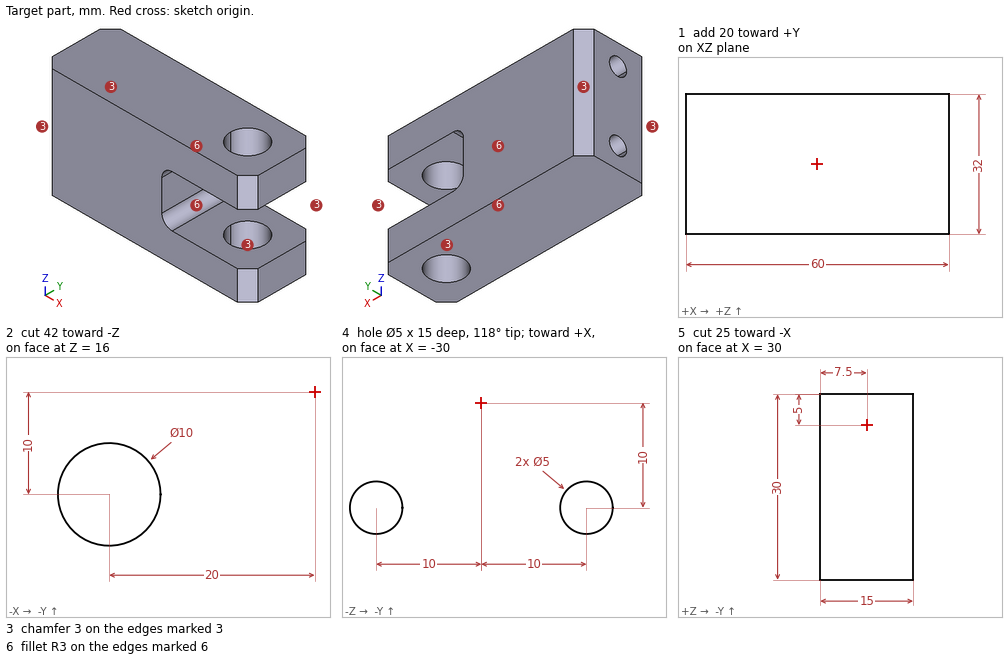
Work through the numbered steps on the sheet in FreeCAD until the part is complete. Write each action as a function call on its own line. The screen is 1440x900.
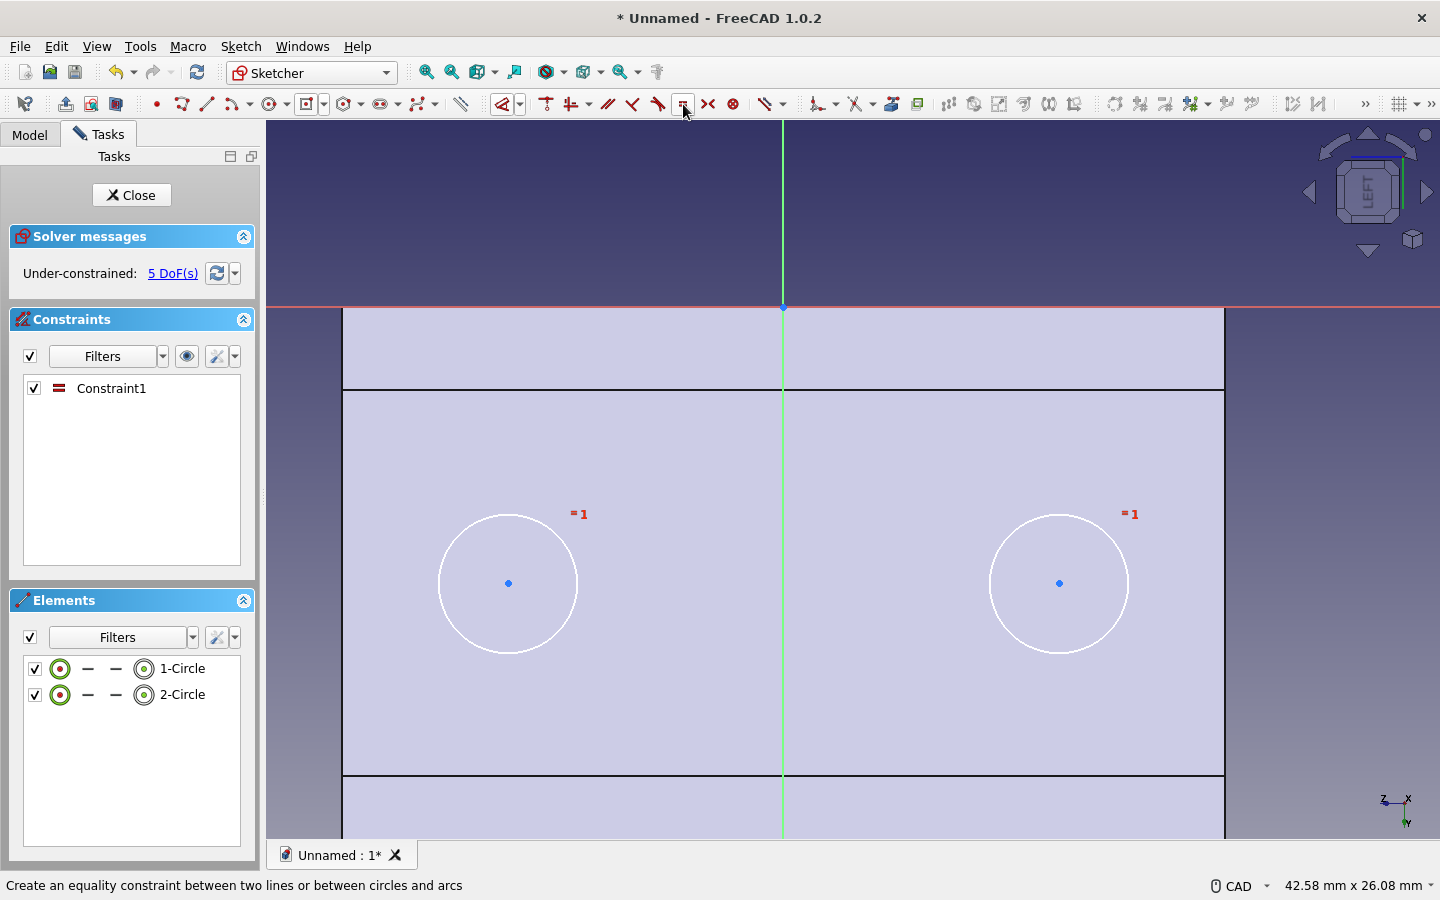
click(1059, 584)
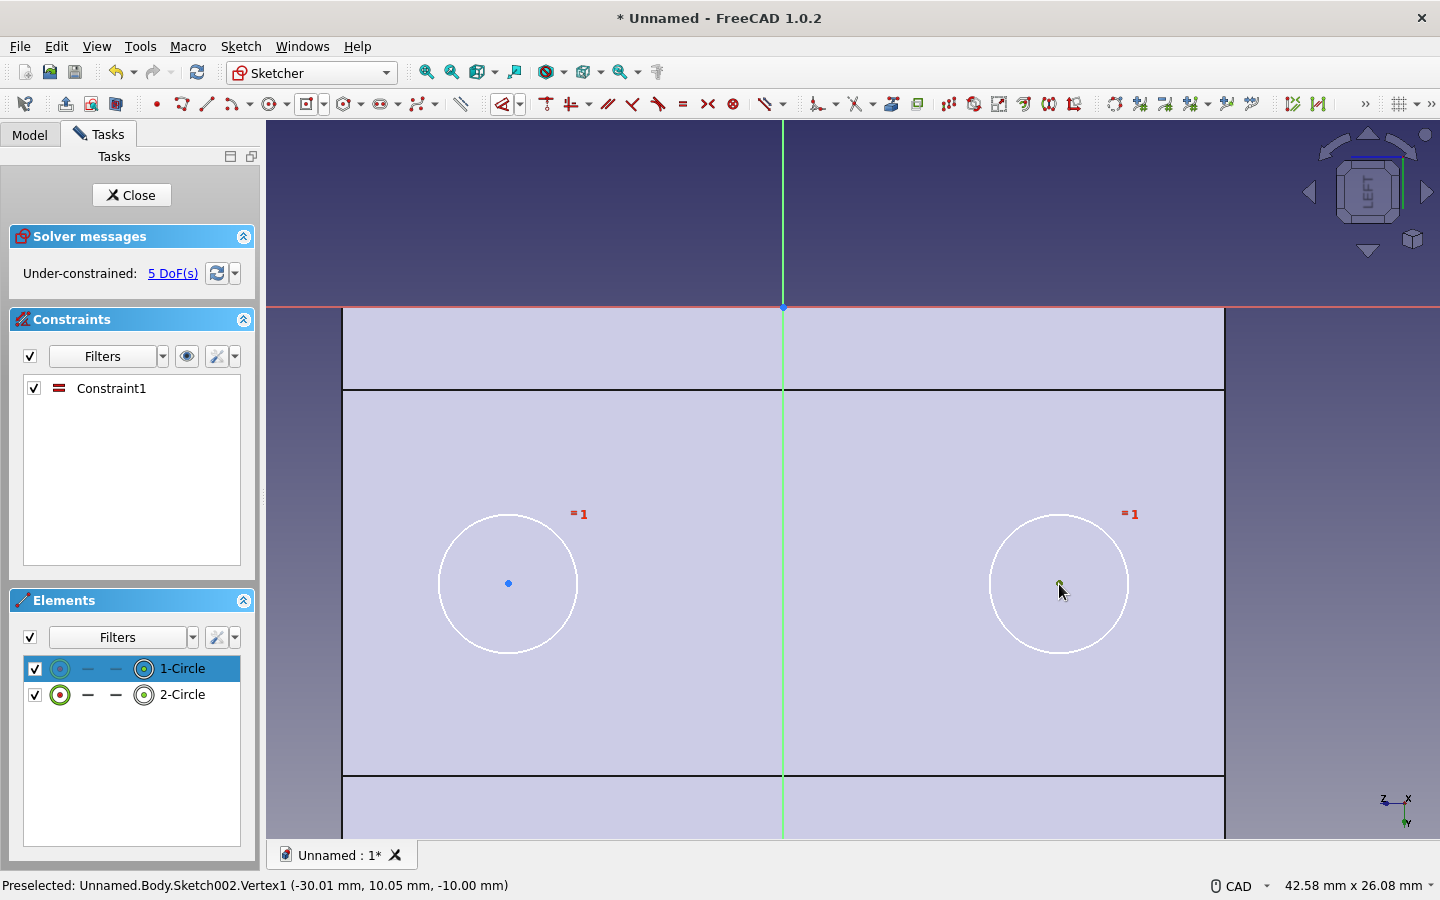
click(508, 584)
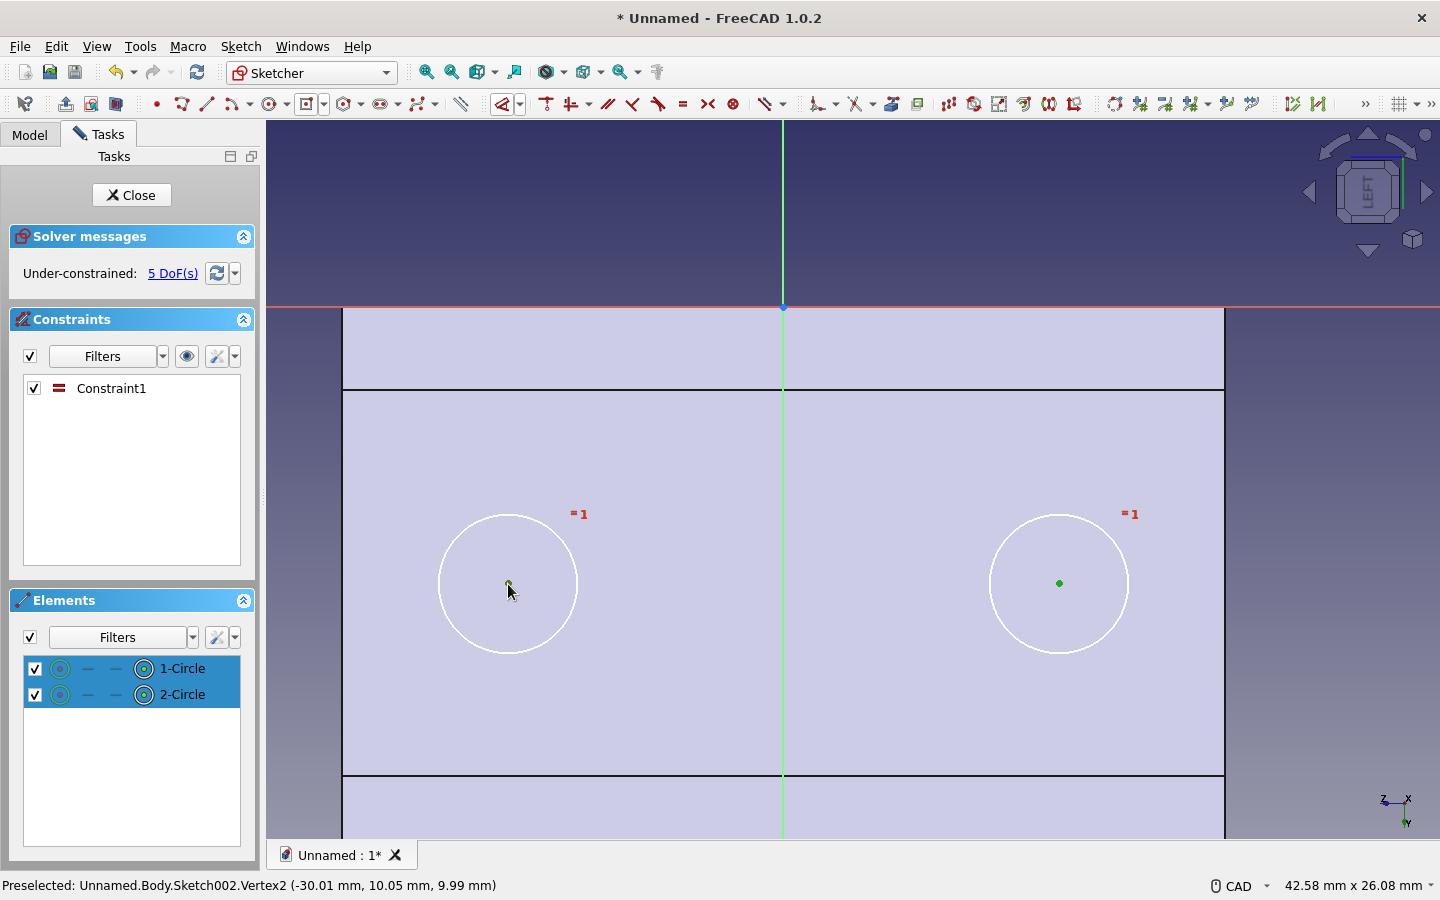
key(h)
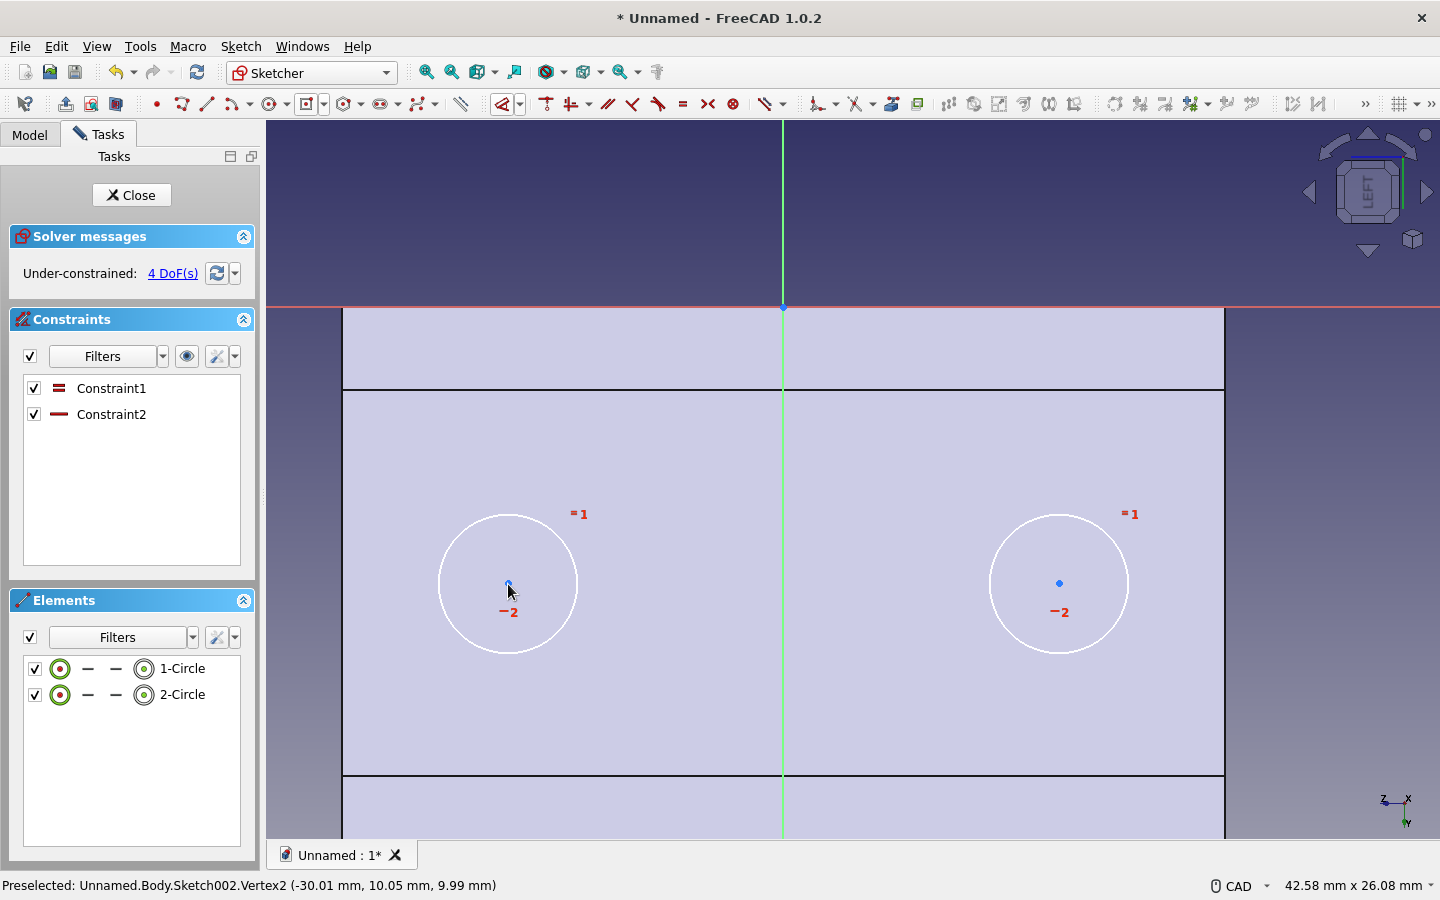
click(1108, 535)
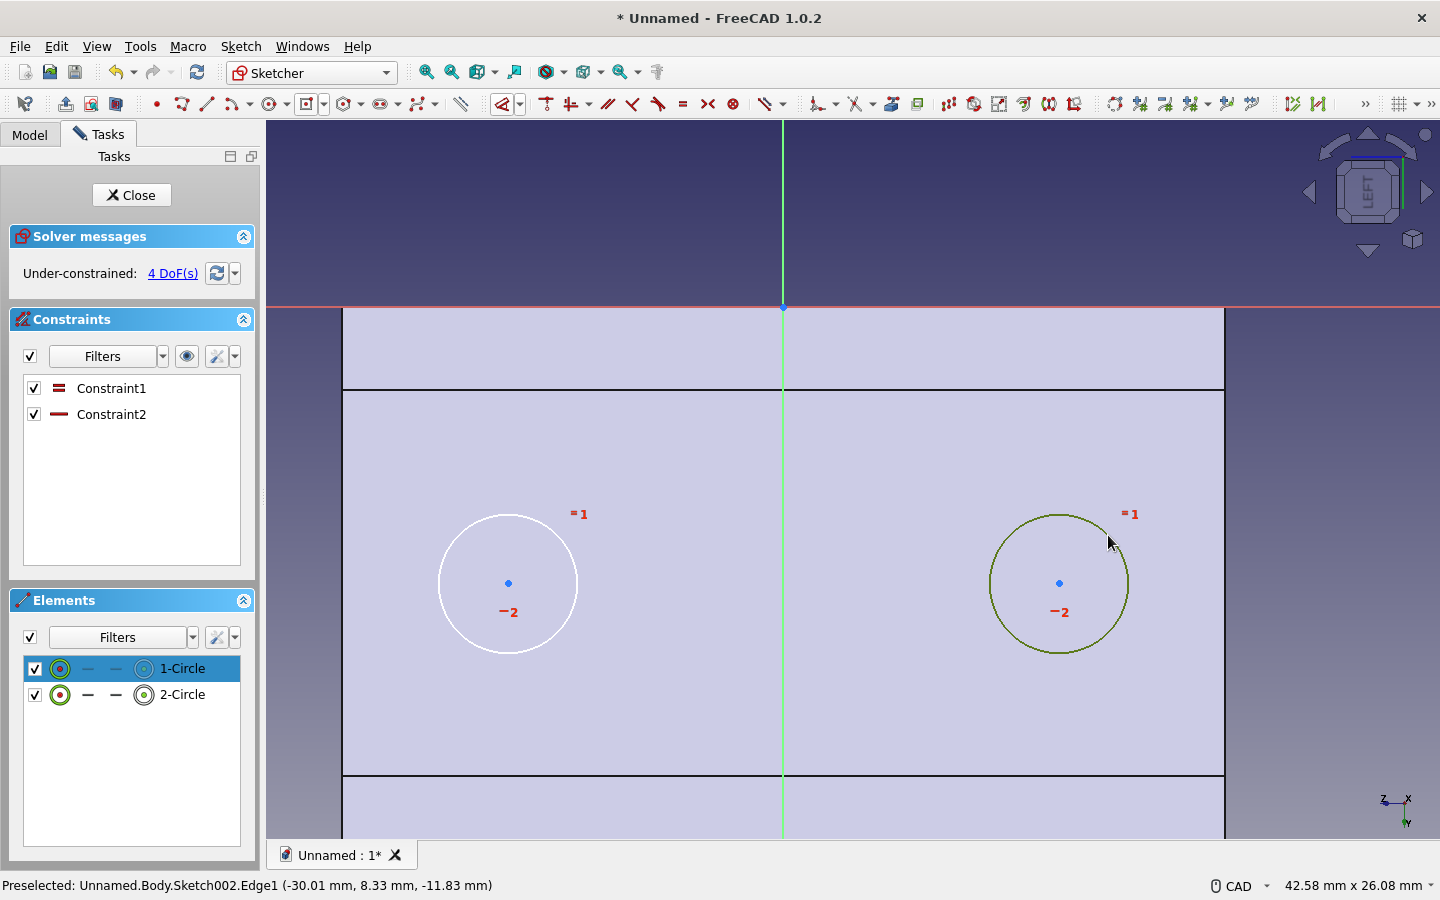
click(520, 104)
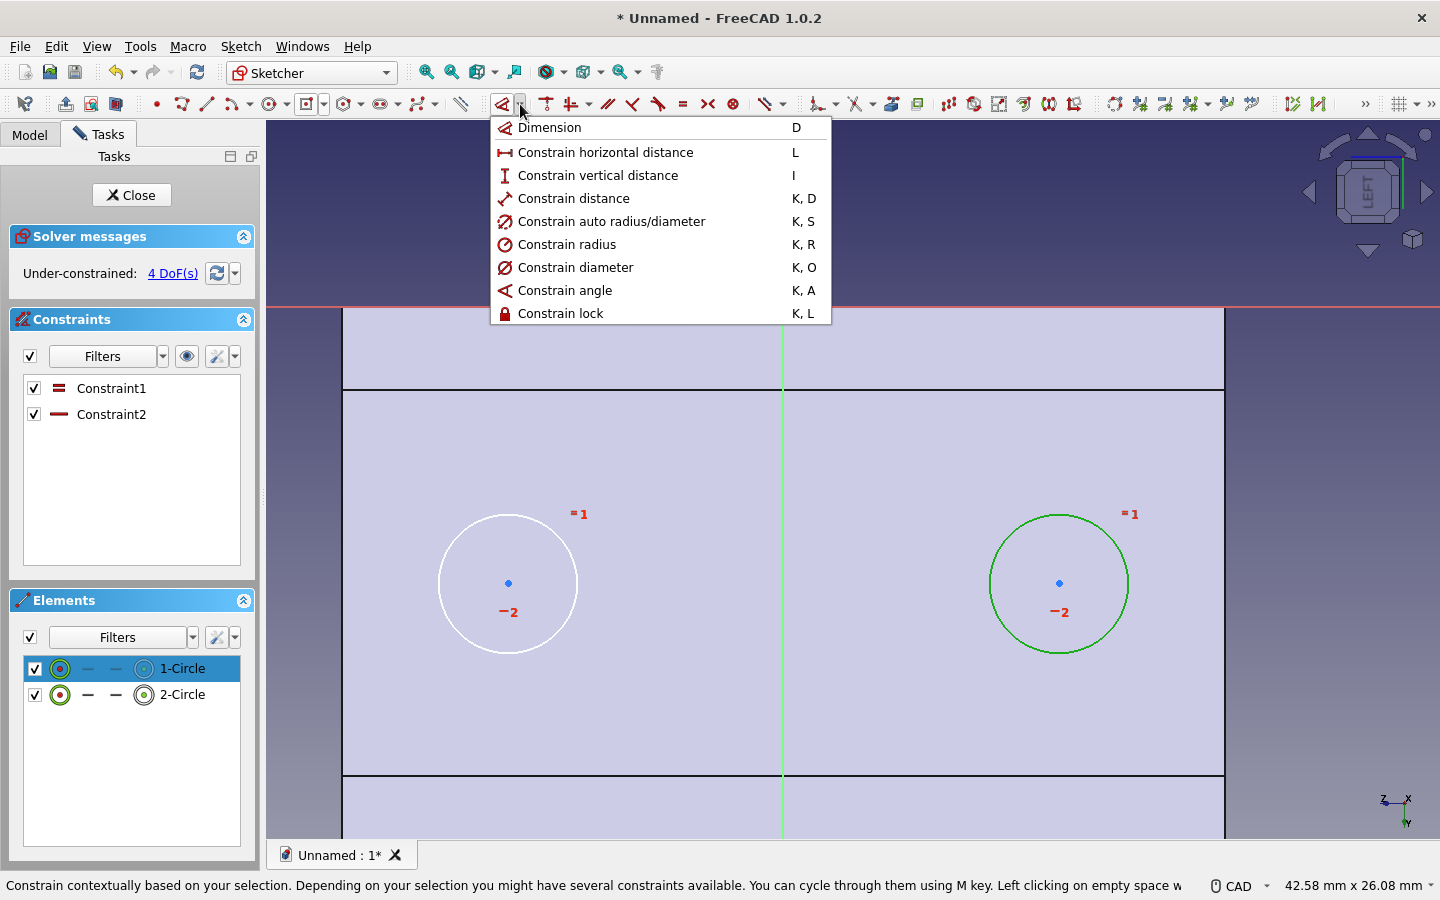
click(661, 268)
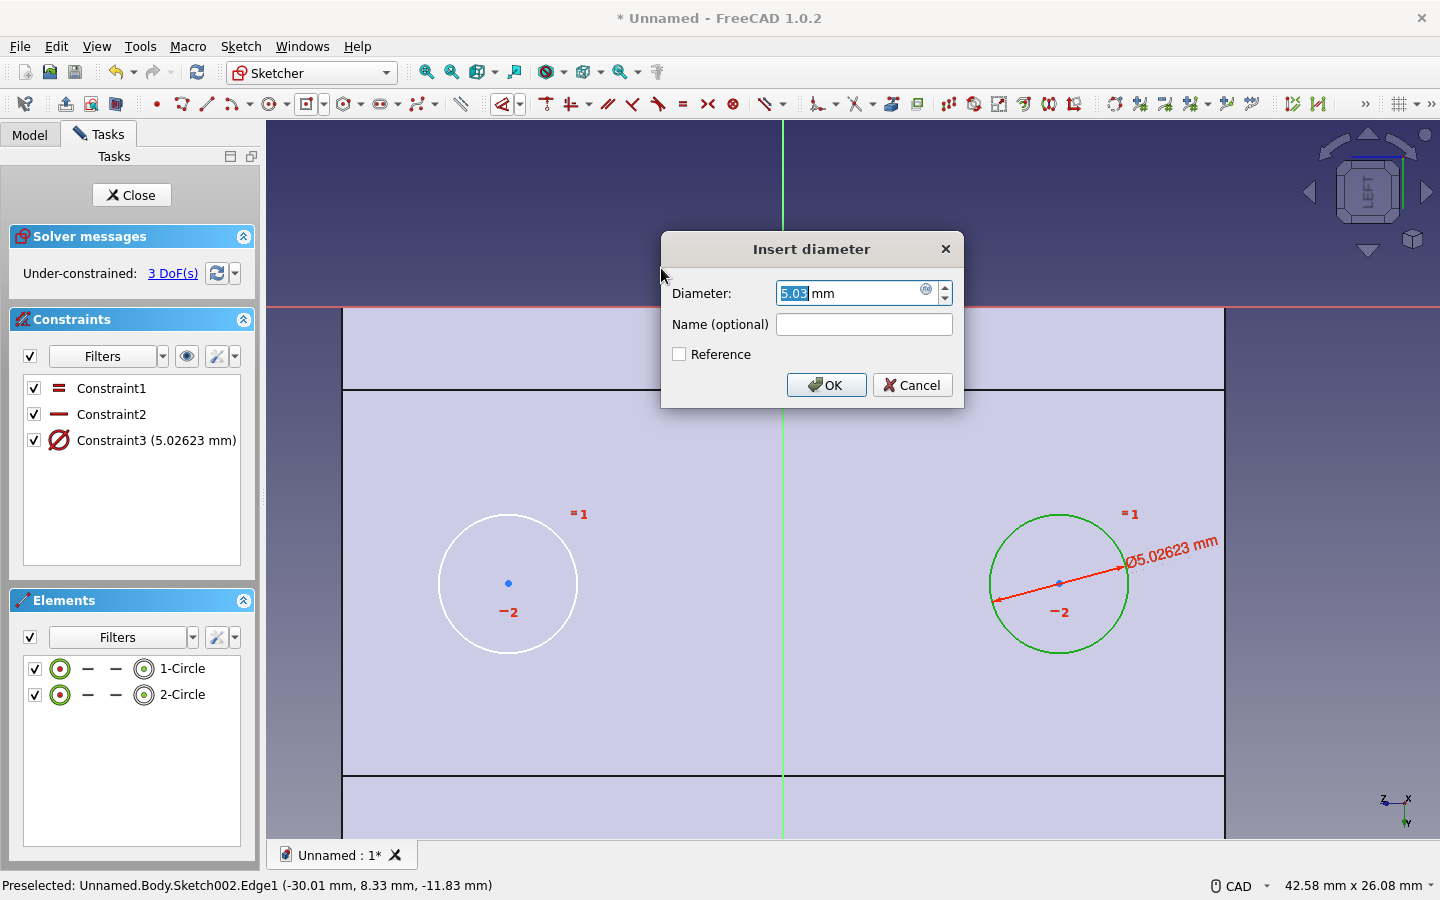
text(5)
key(Return)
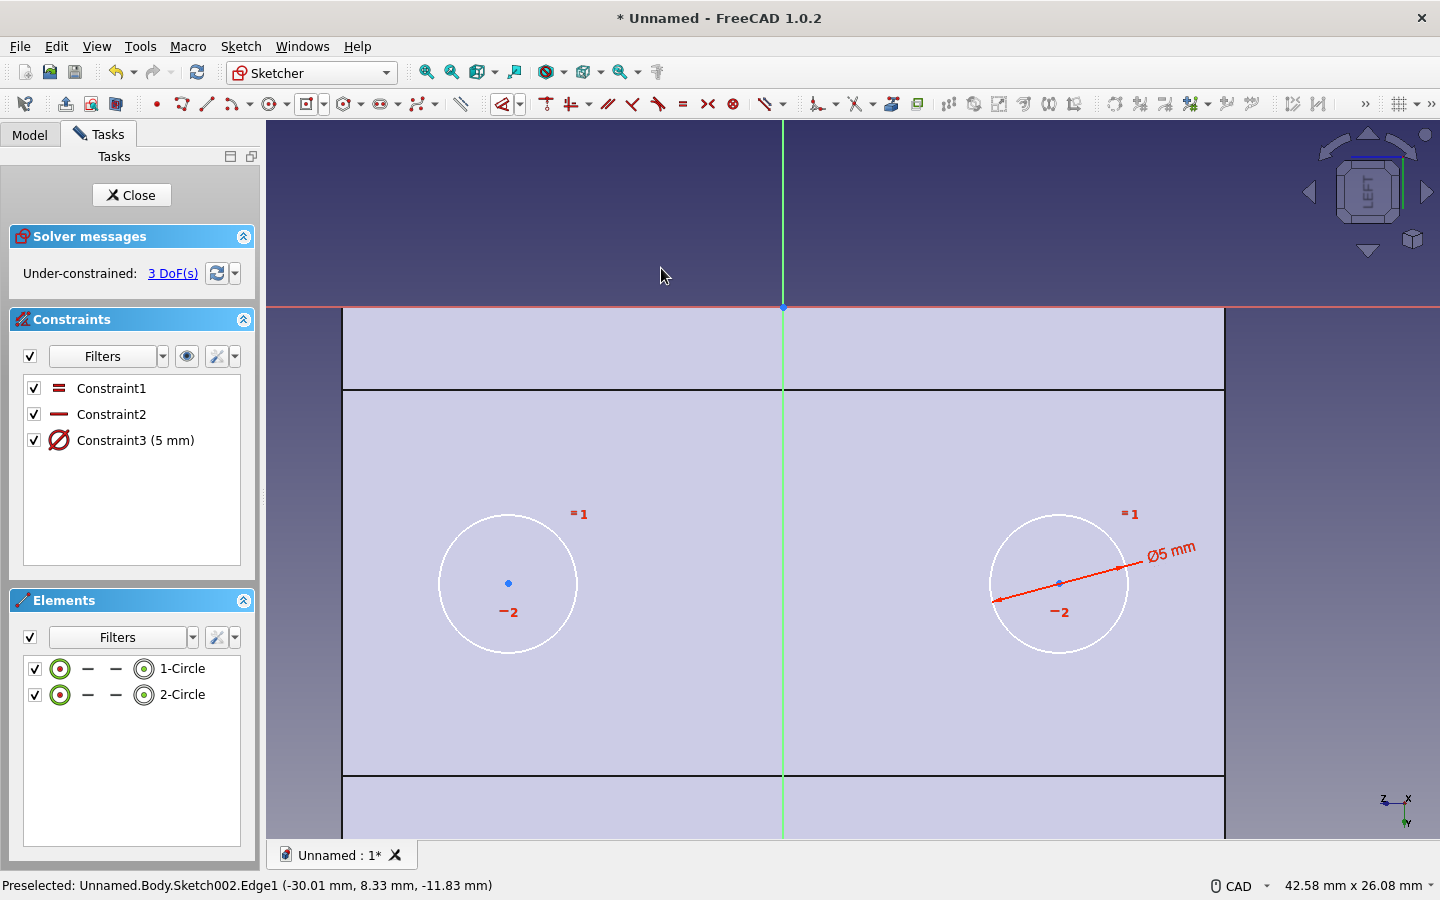
click(1059, 584)